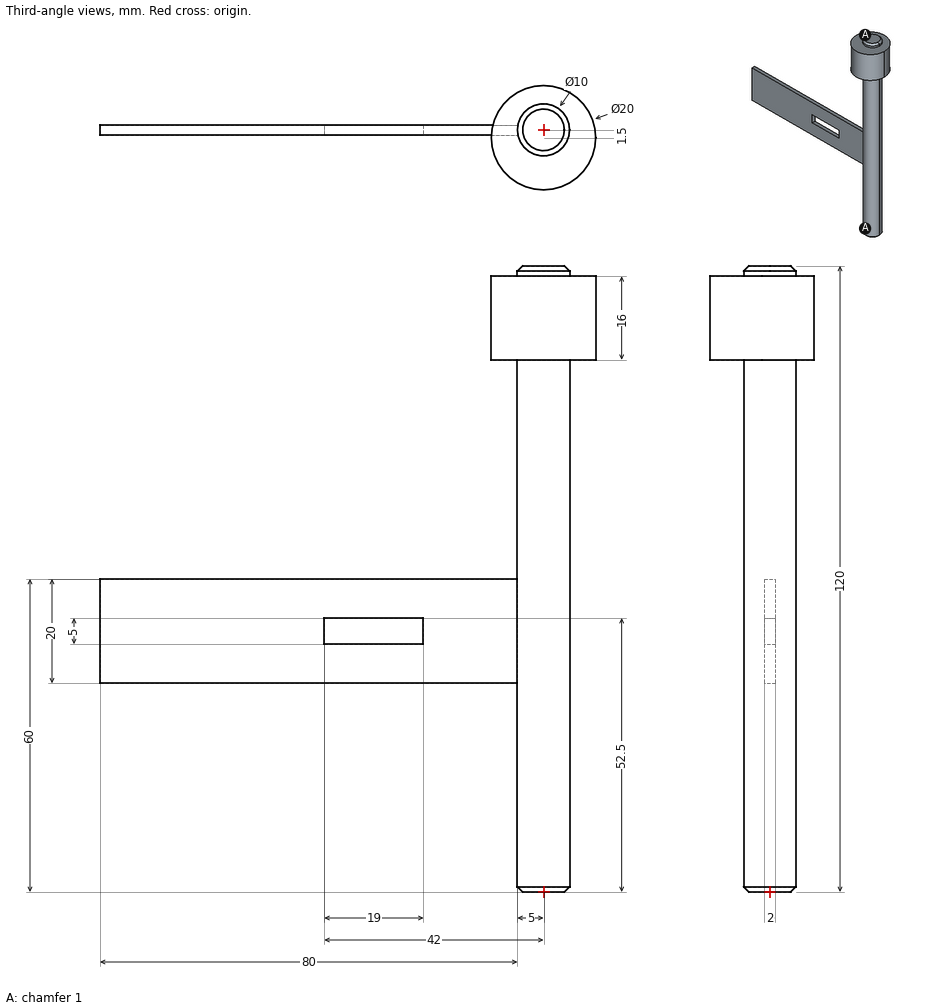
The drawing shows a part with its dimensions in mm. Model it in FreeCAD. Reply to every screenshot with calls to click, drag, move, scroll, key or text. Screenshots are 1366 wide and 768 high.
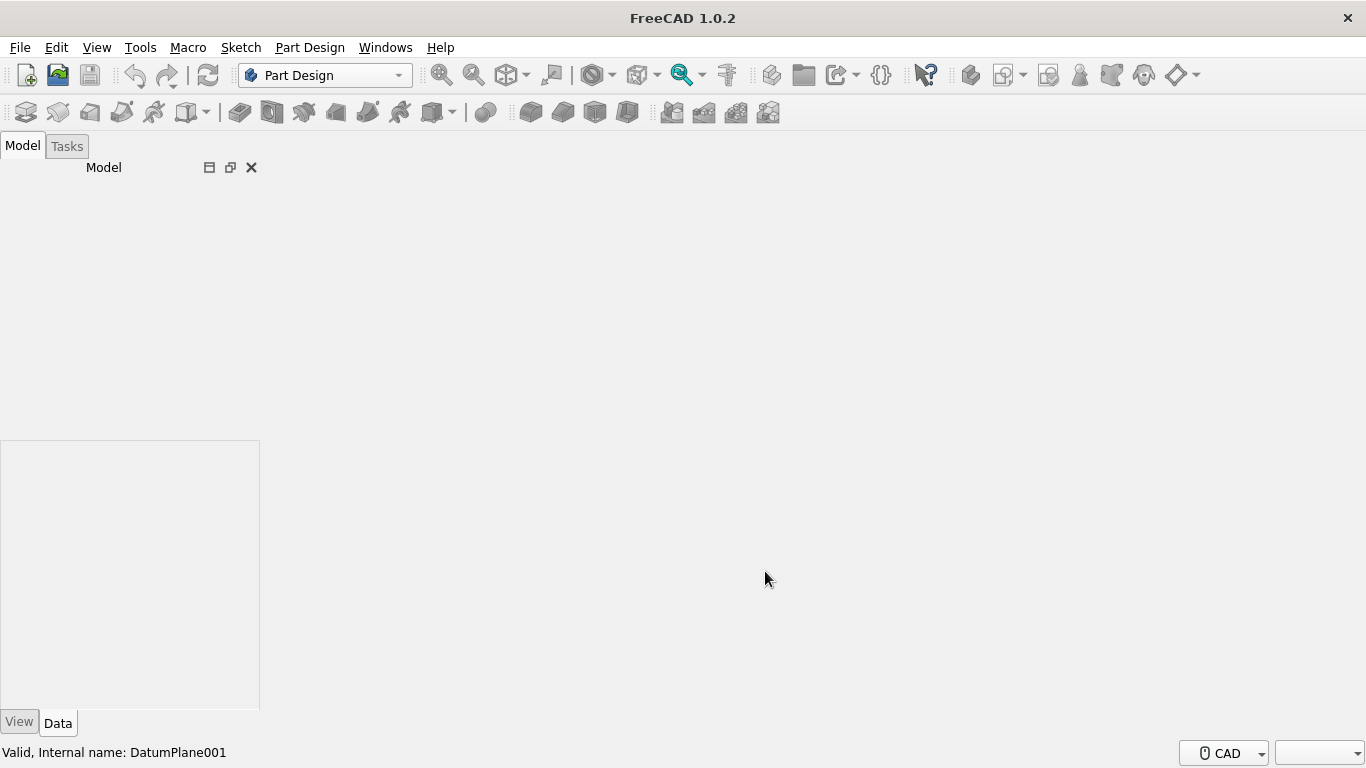
click(26, 76)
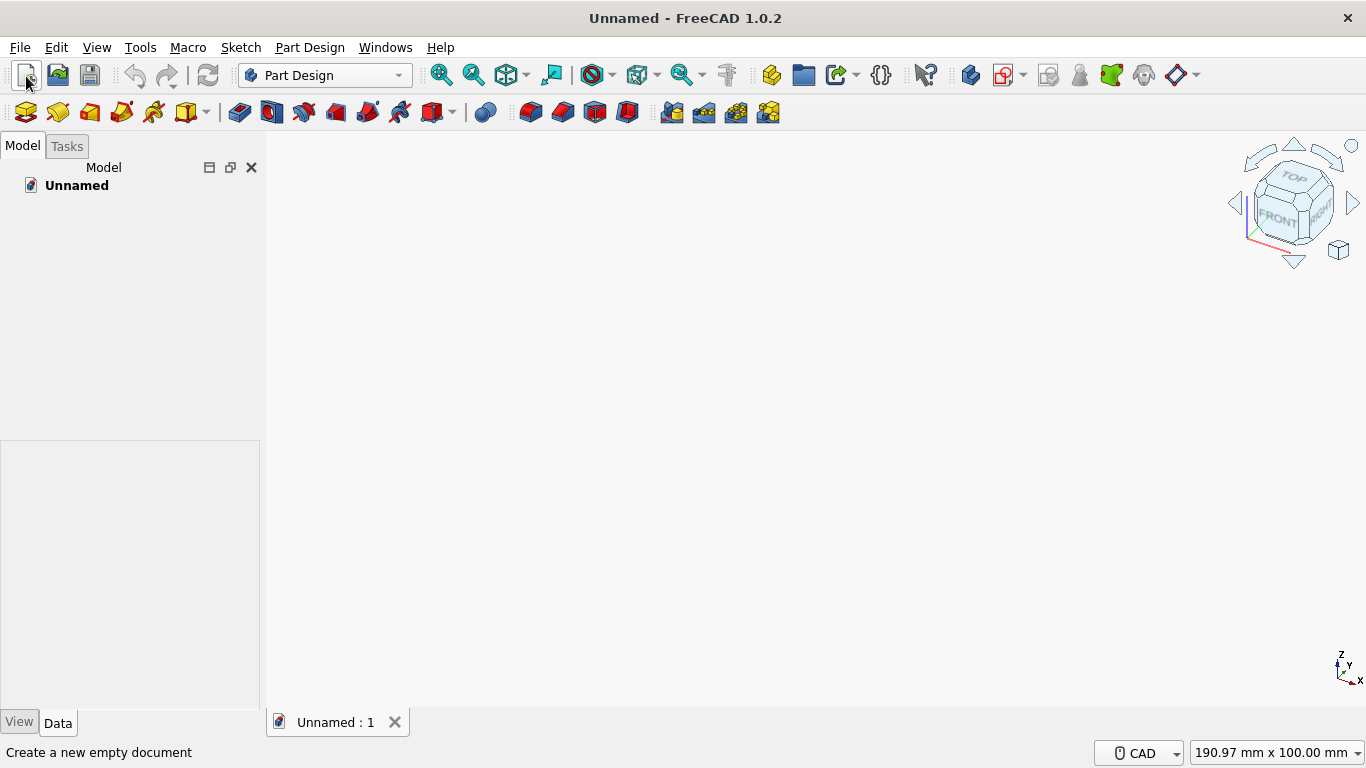
click(1004, 76)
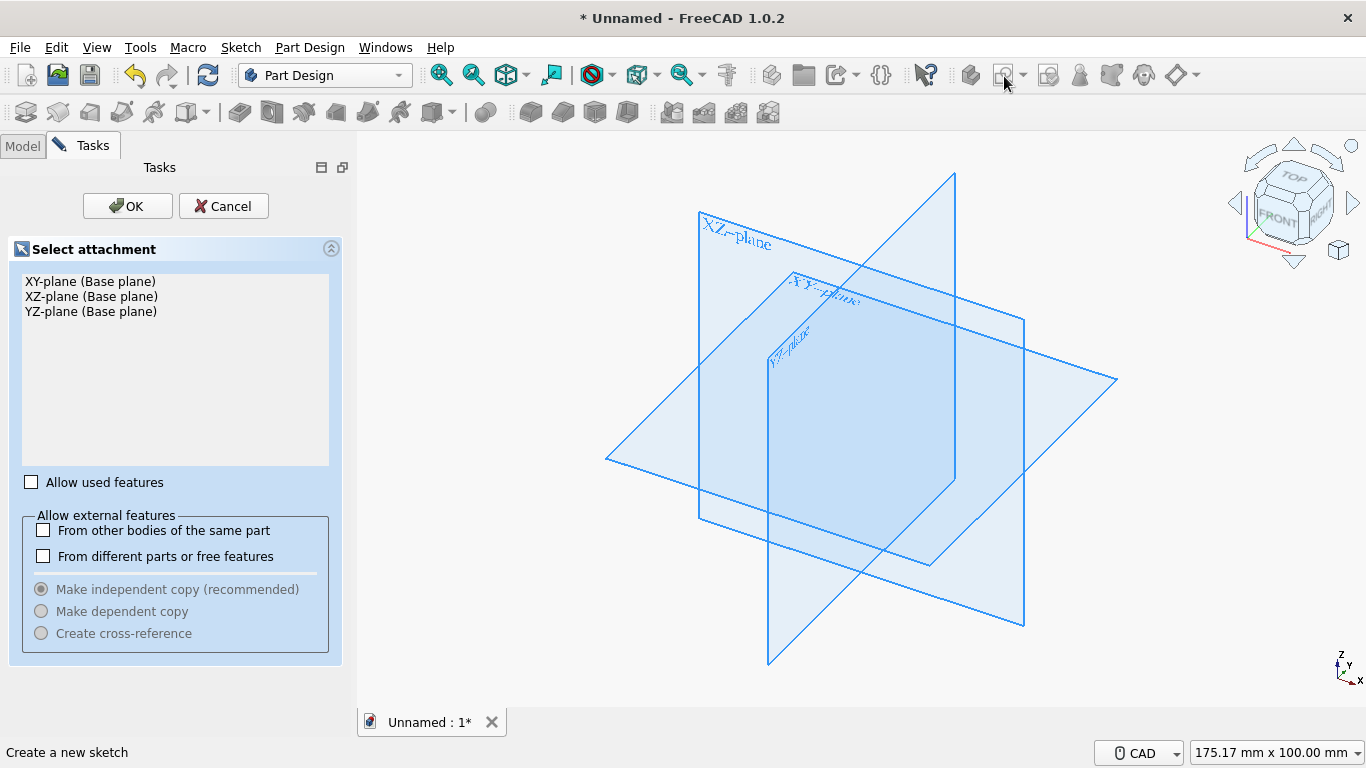
click(82, 282)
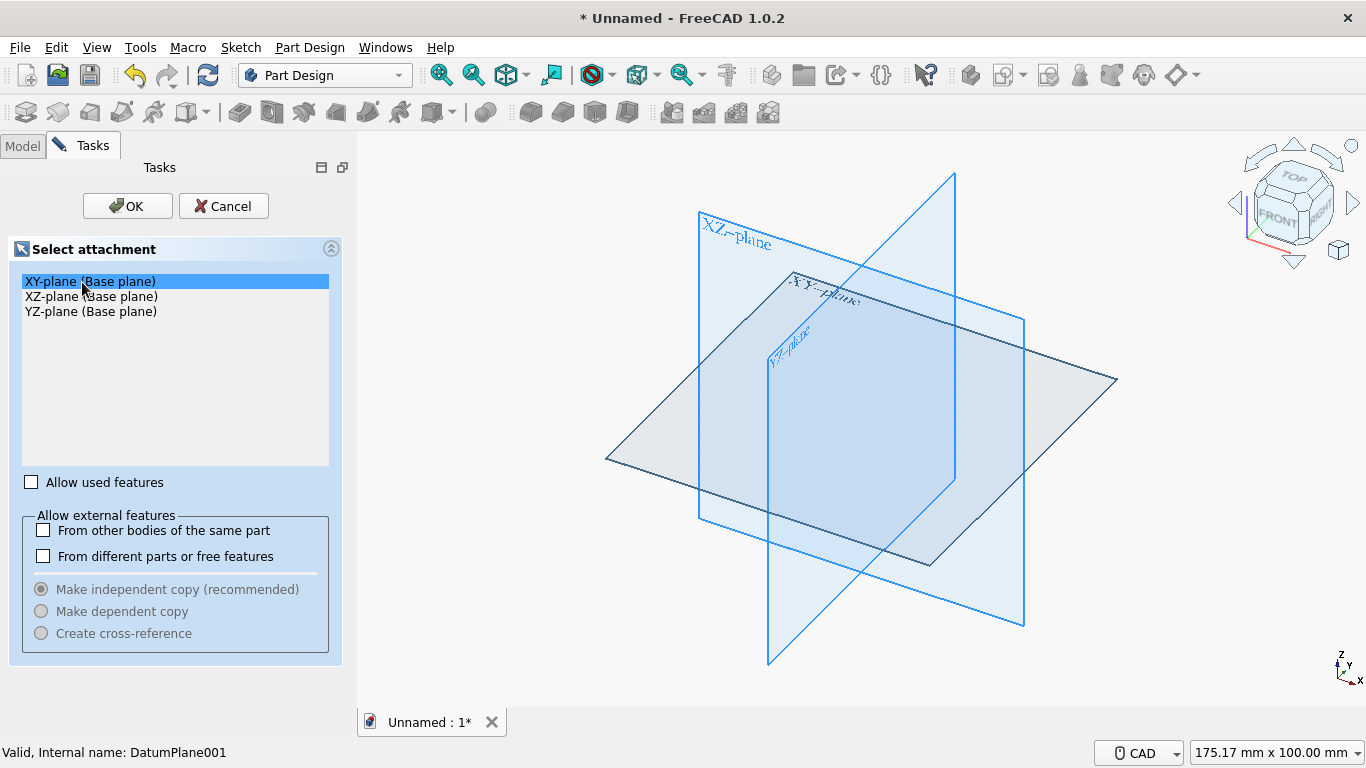
click(128, 206)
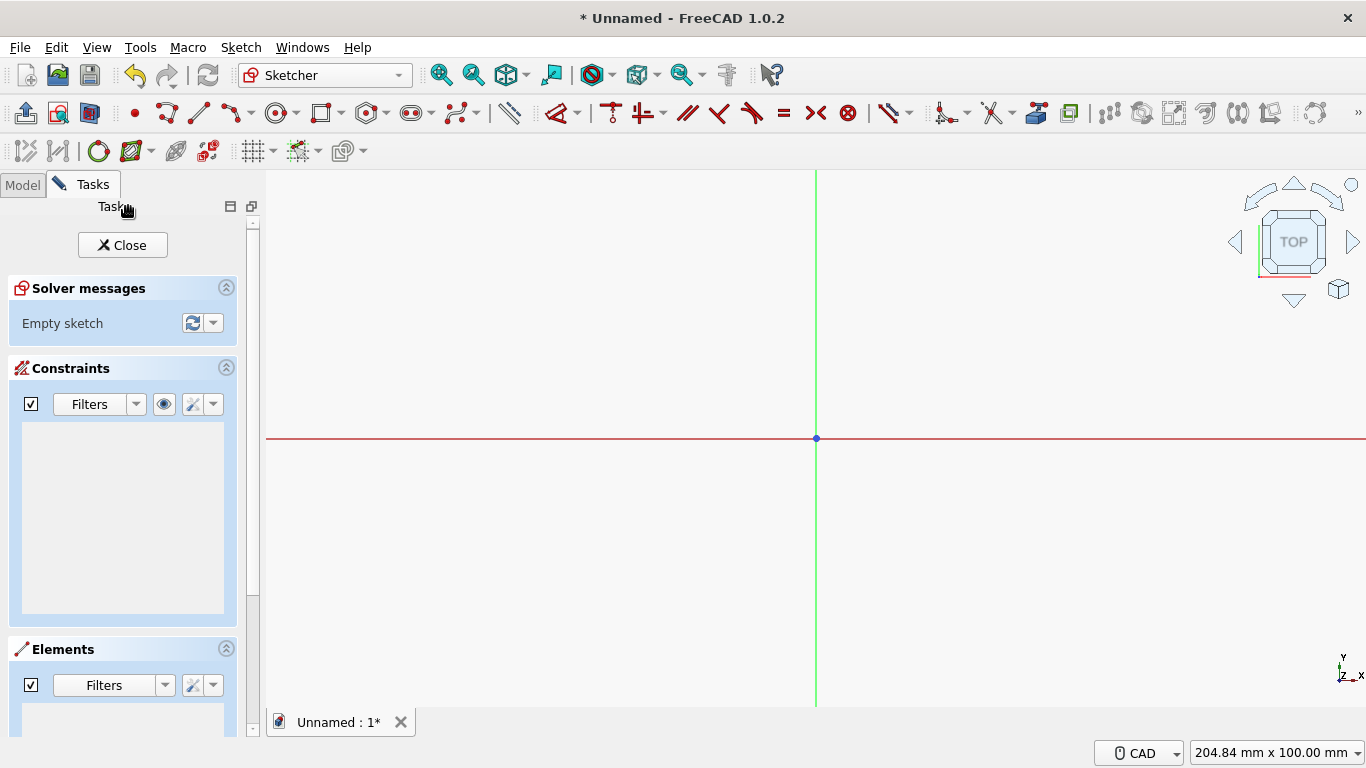
scroll(830, 438, up, 9)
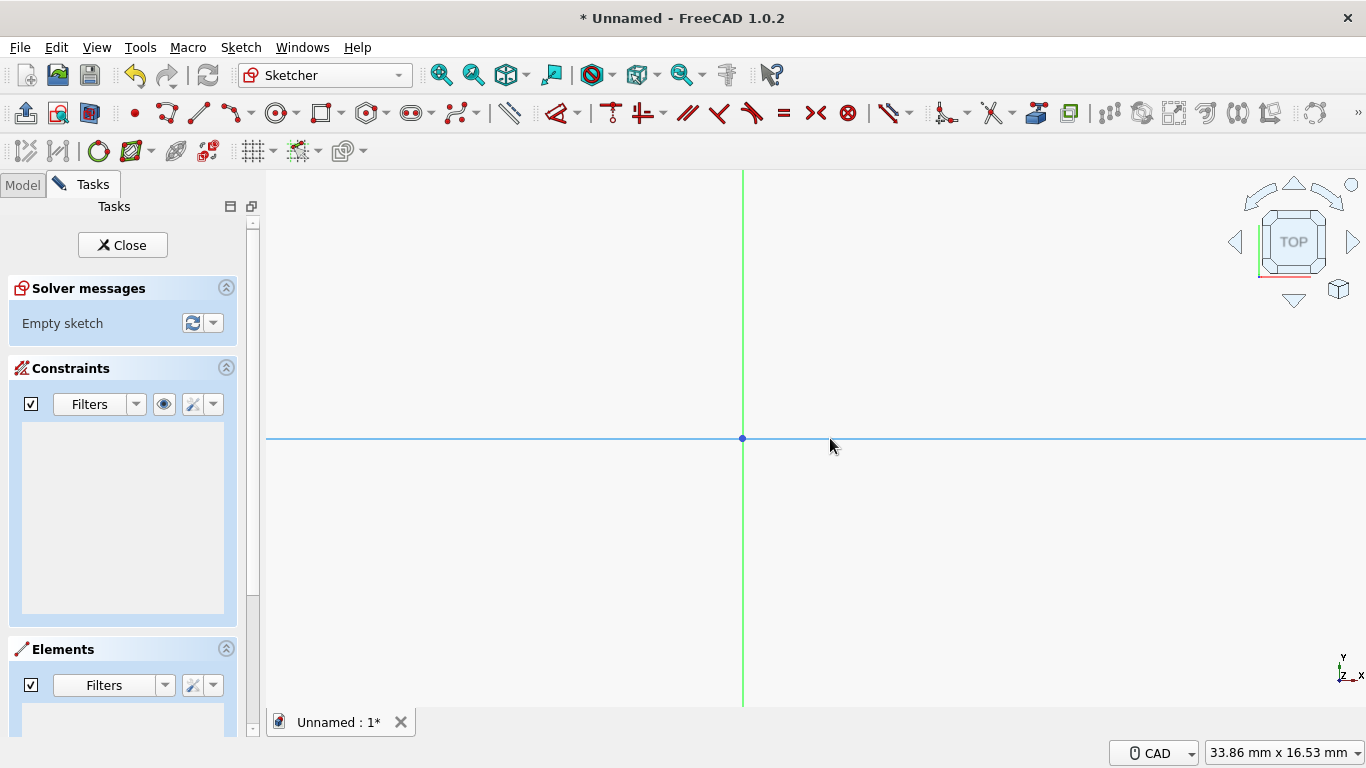
click(276, 114)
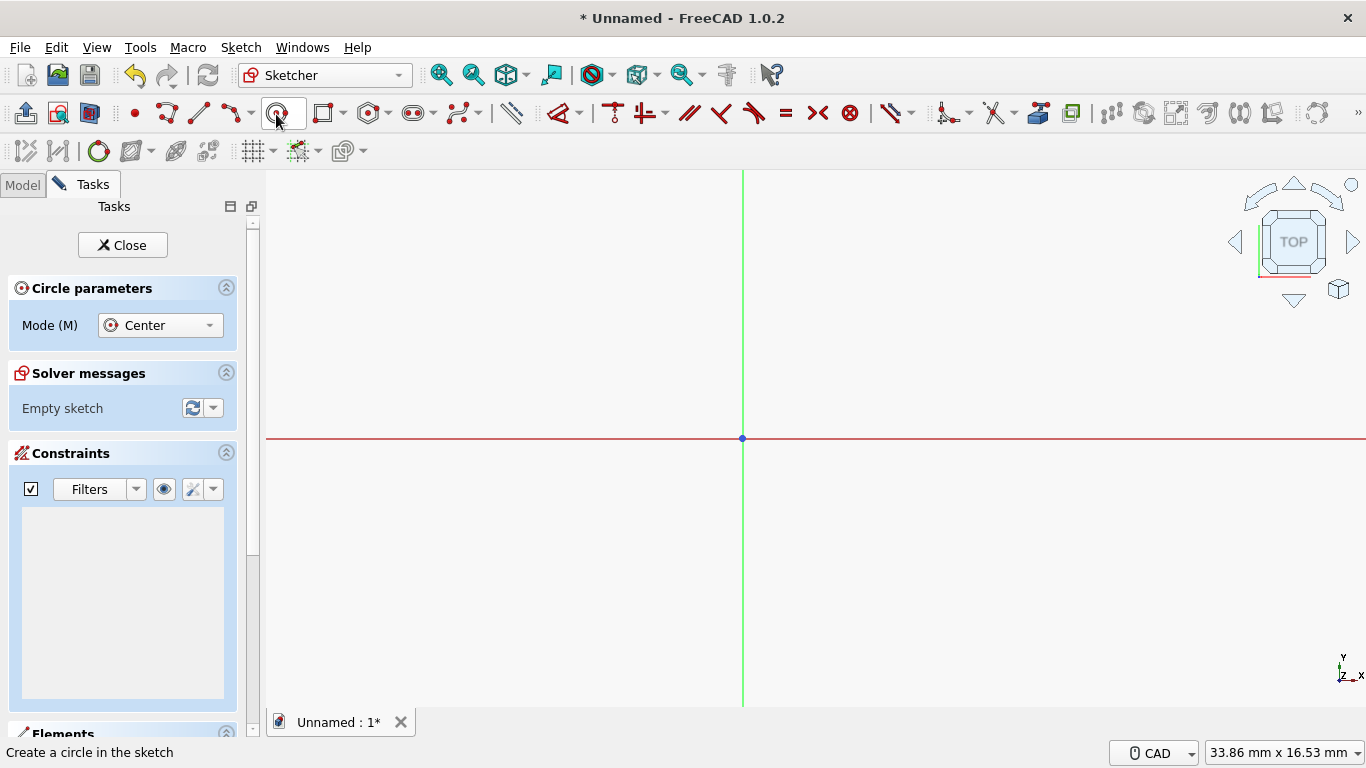
click(743, 438)
click(858, 324)
key(Escape)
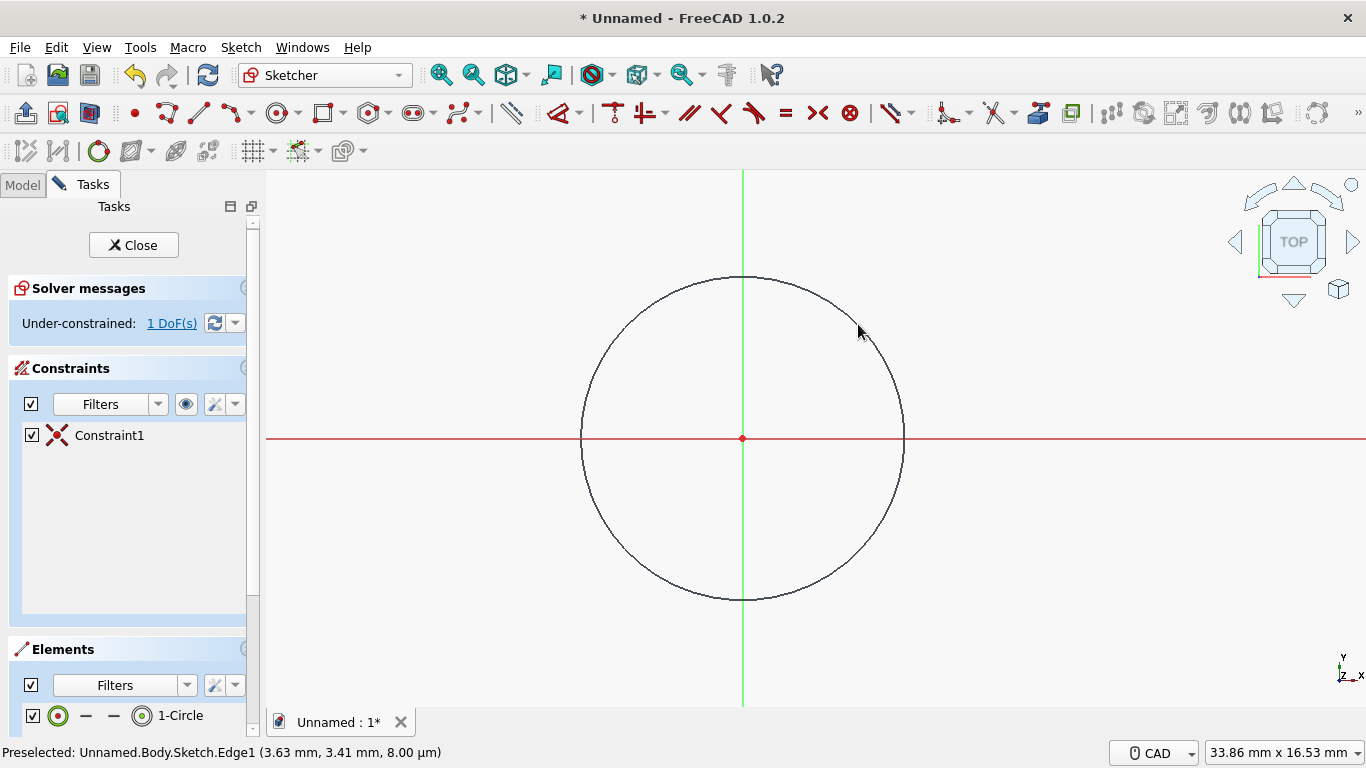
click(857, 324)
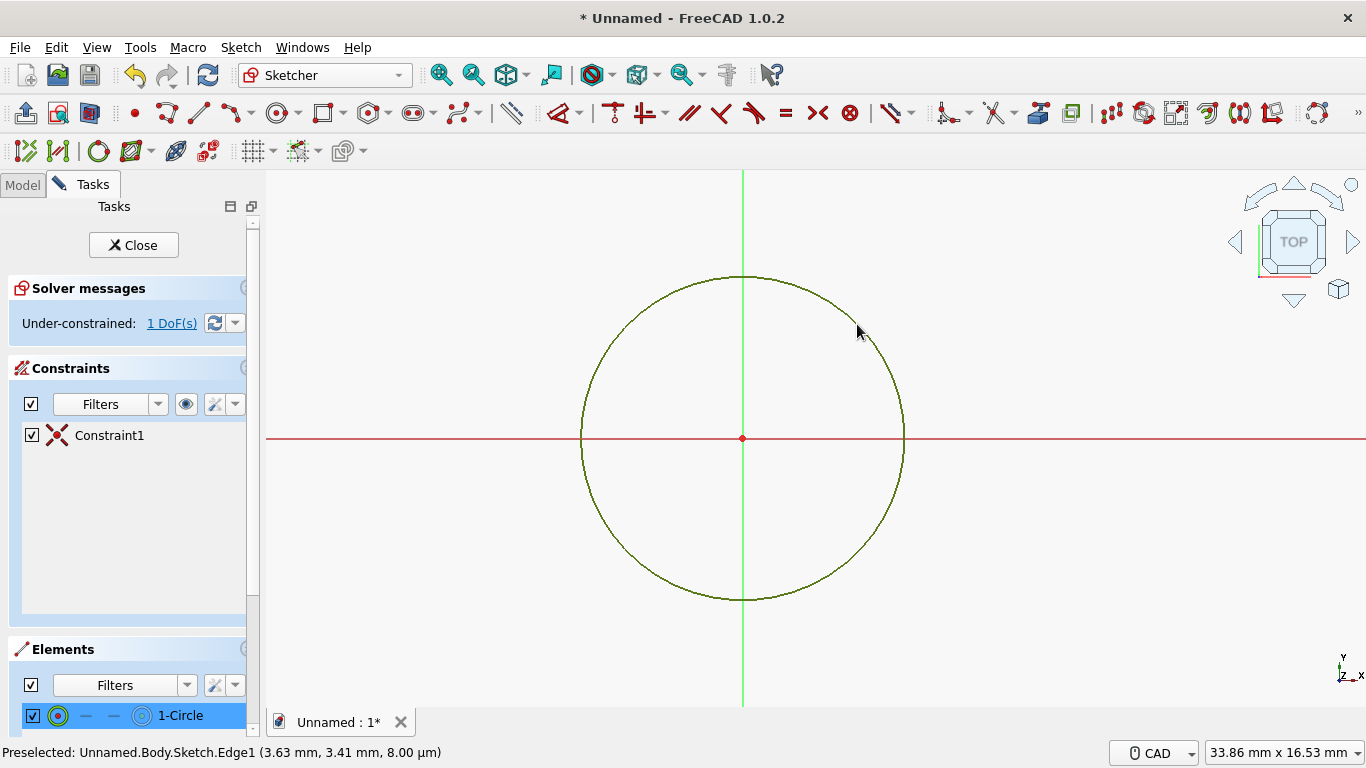
click(582, 114)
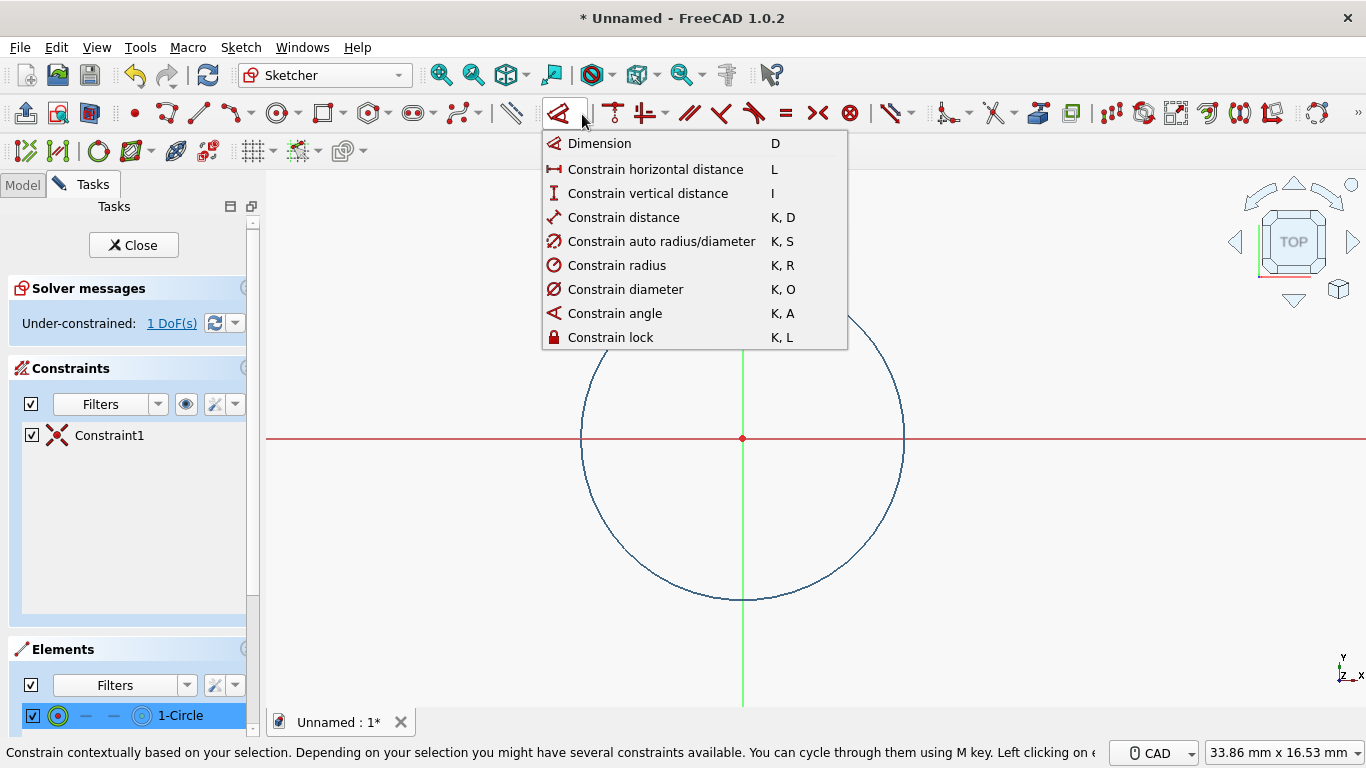
click(695, 289)